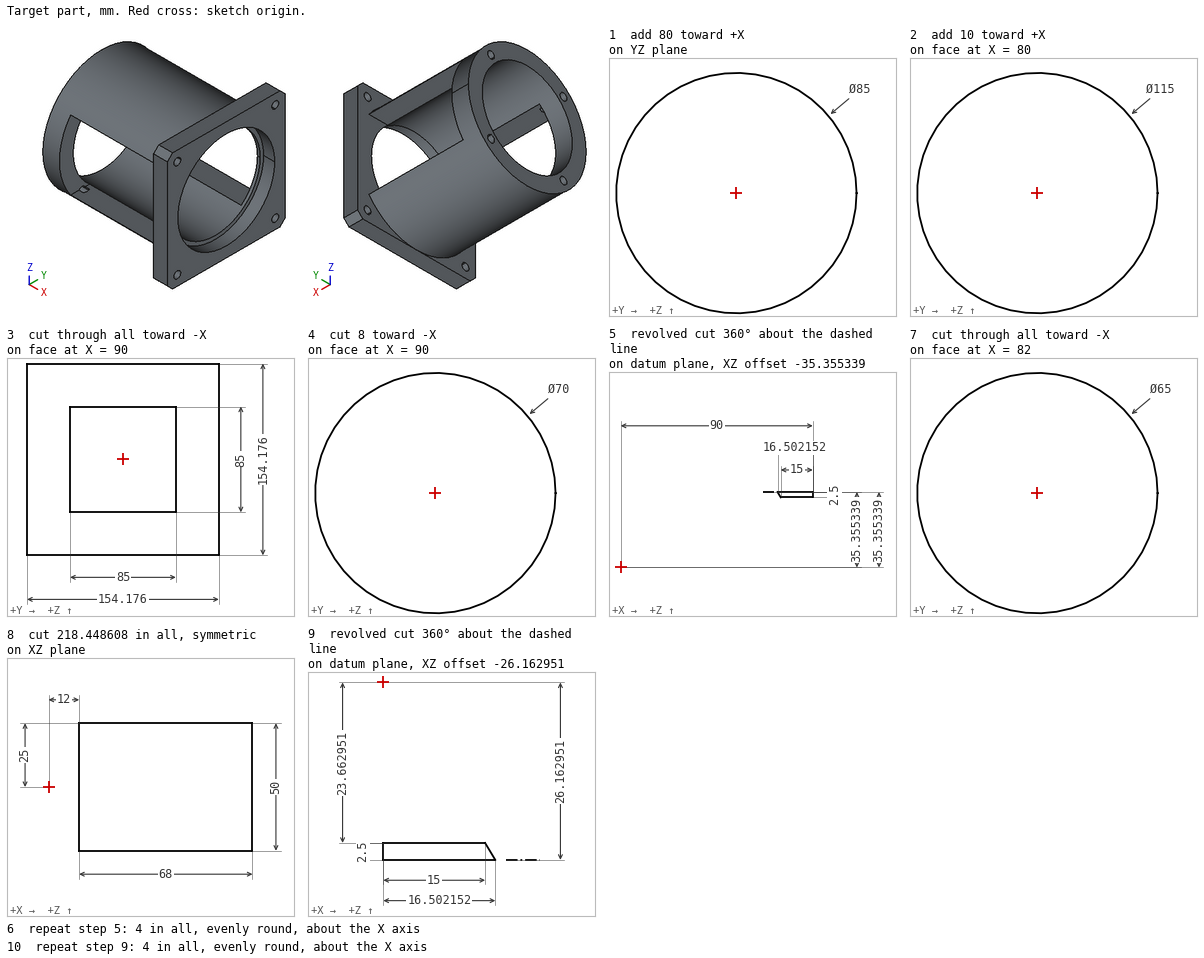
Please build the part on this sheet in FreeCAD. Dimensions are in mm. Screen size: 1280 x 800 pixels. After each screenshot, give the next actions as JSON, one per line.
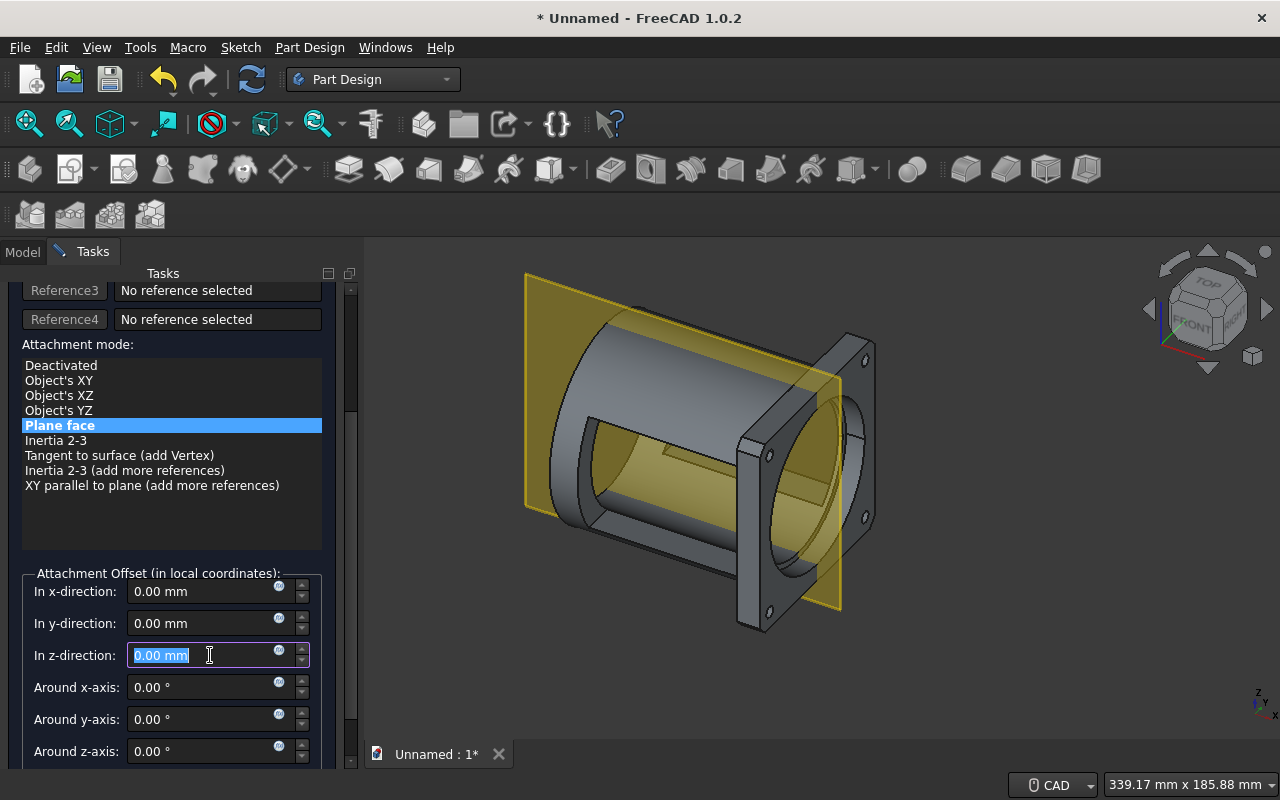
{"action": "type", "text": "-26.162951"}
{"action": "key", "text": "Tab"}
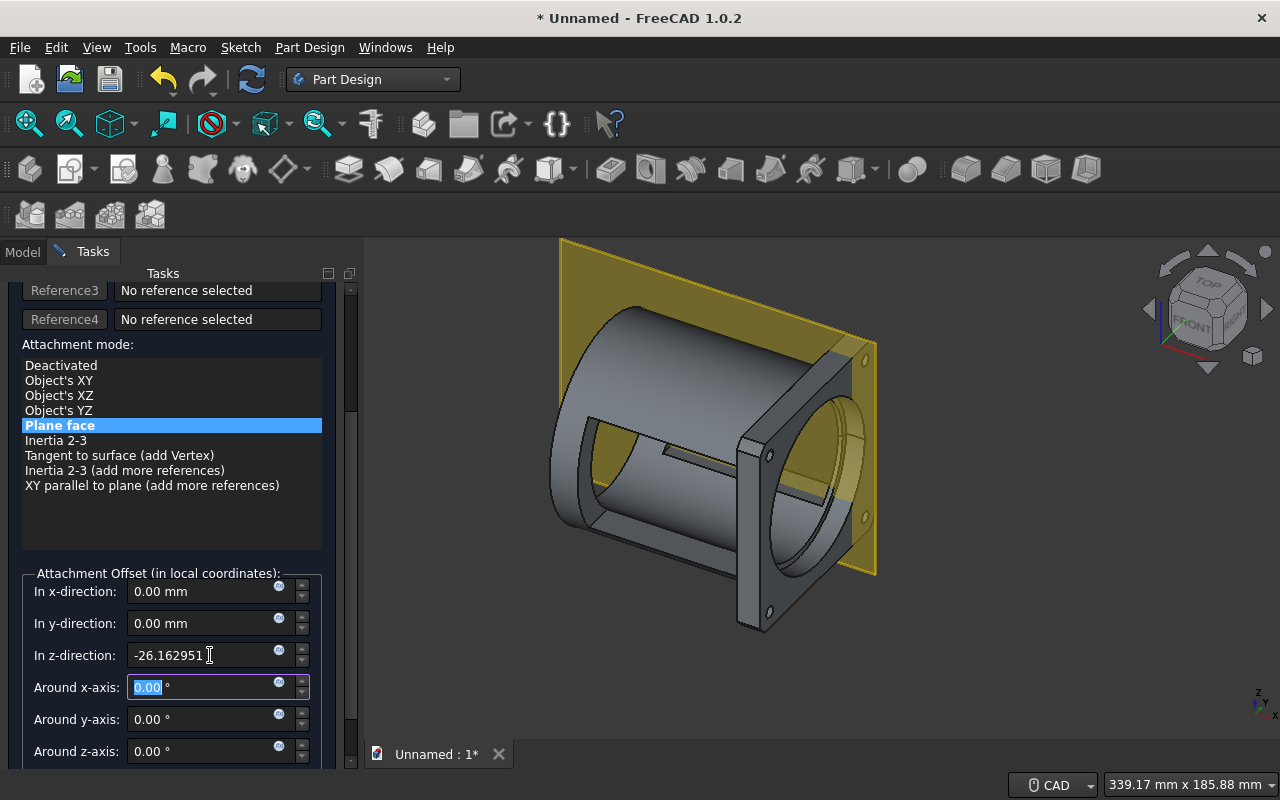
{"action": "scroll", "coordinate": [351, 526], "scroll_direction": "up", "scroll_amount": 4}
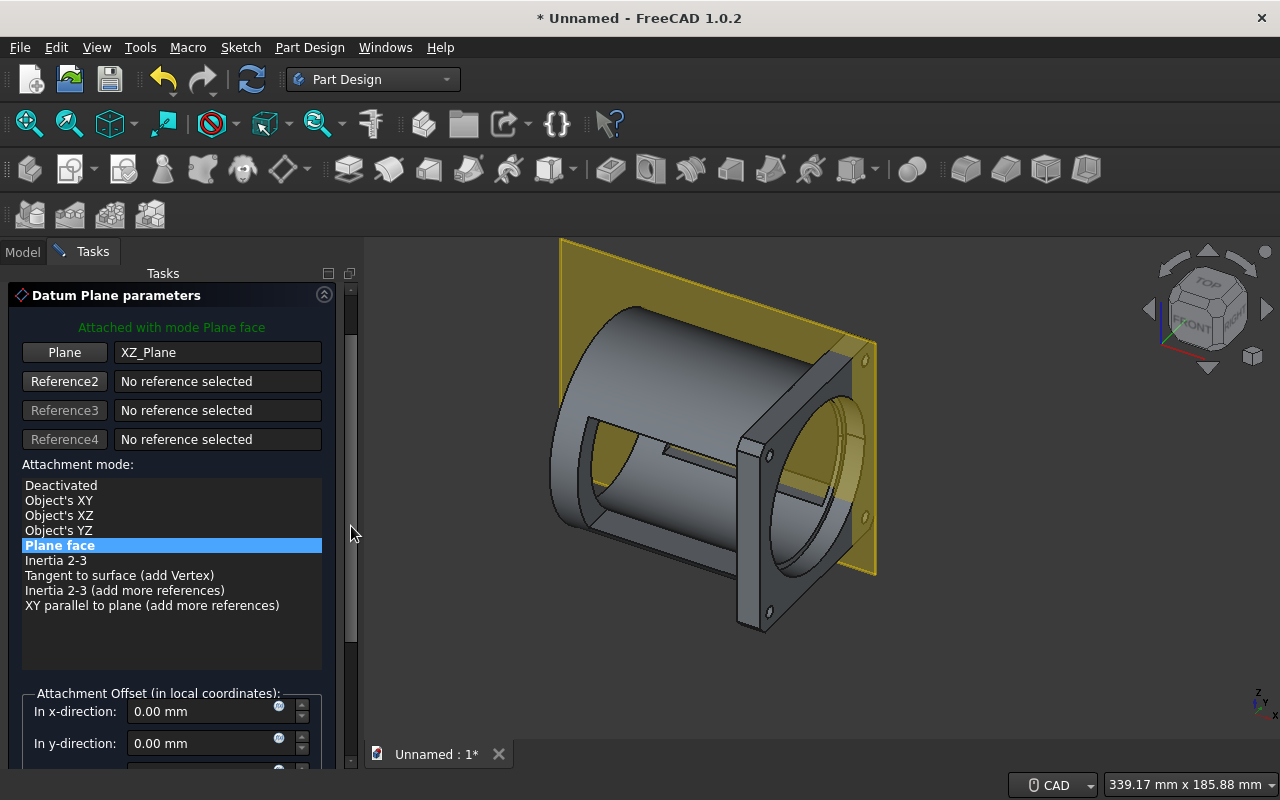
{"action": "left_click", "coordinate": [124, 312]}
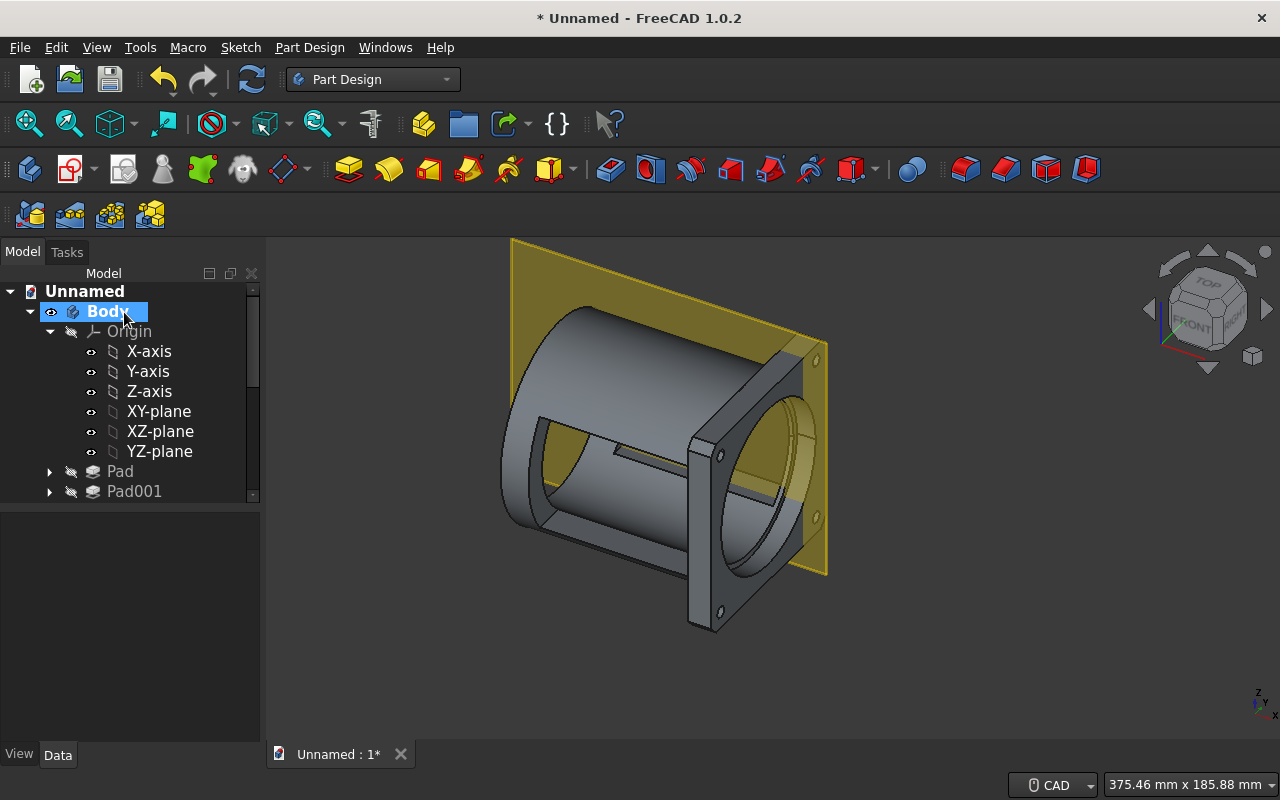
{"action": "scroll", "coordinate": [100, 387], "scroll_direction": "down", "scroll_amount": 3}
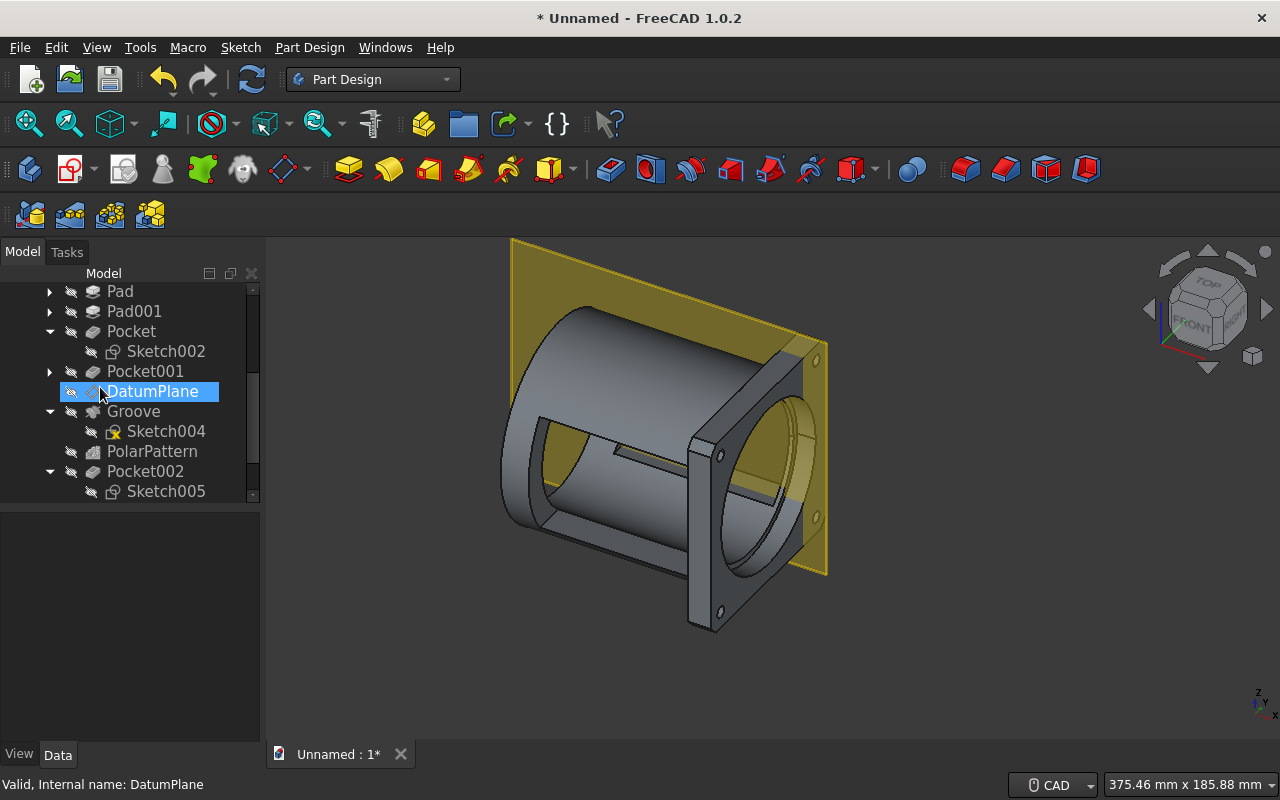
{"action": "scroll", "coordinate": [140, 387], "scroll_direction": "up", "scroll_amount": 15}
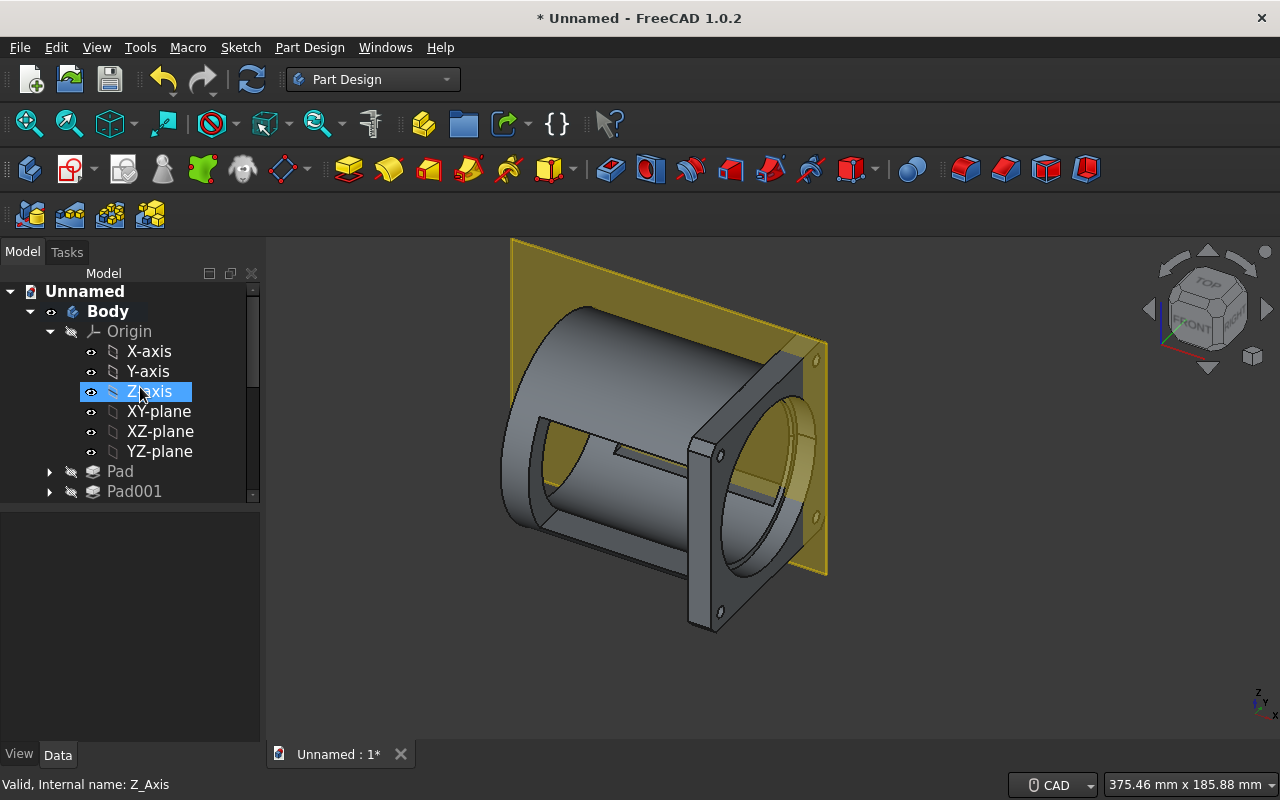
{"action": "scroll", "coordinate": [100, 387], "scroll_direction": "down", "scroll_amount": 6}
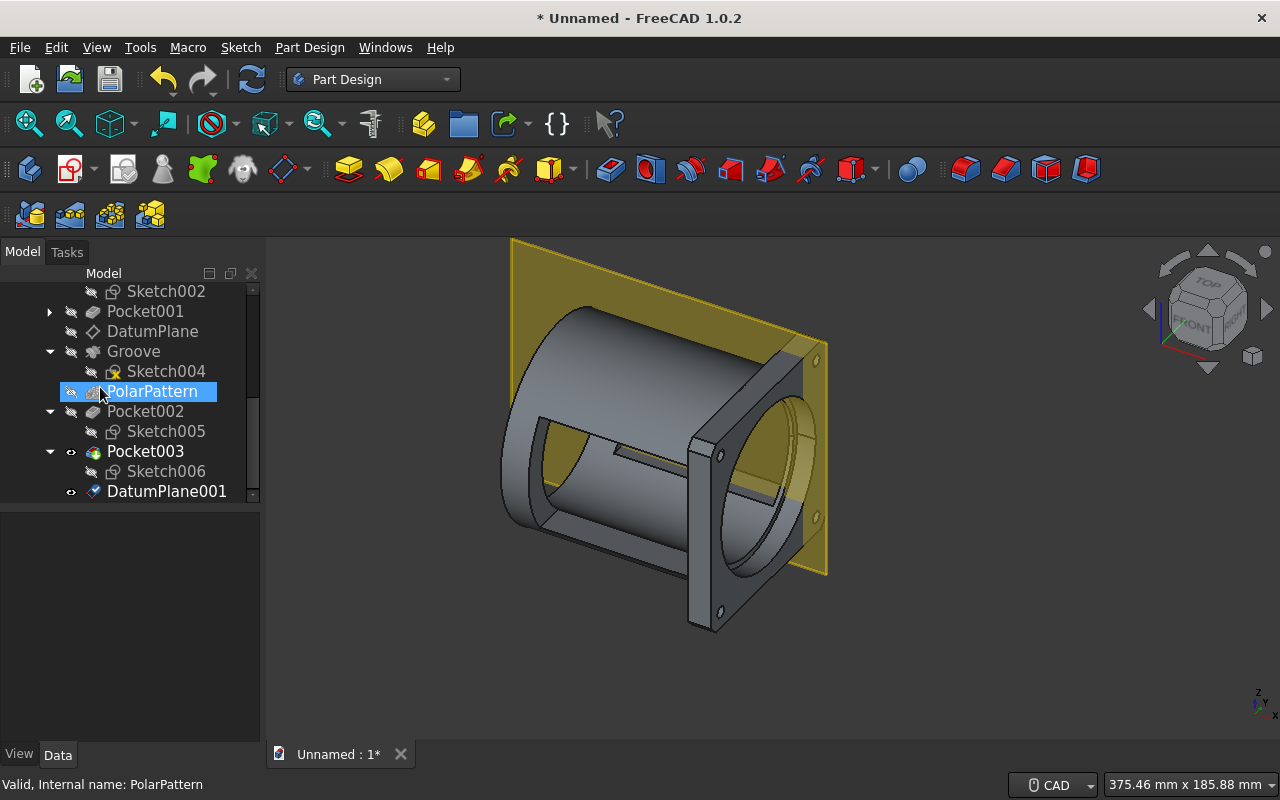
{"action": "left_click", "coordinate": [116, 492]}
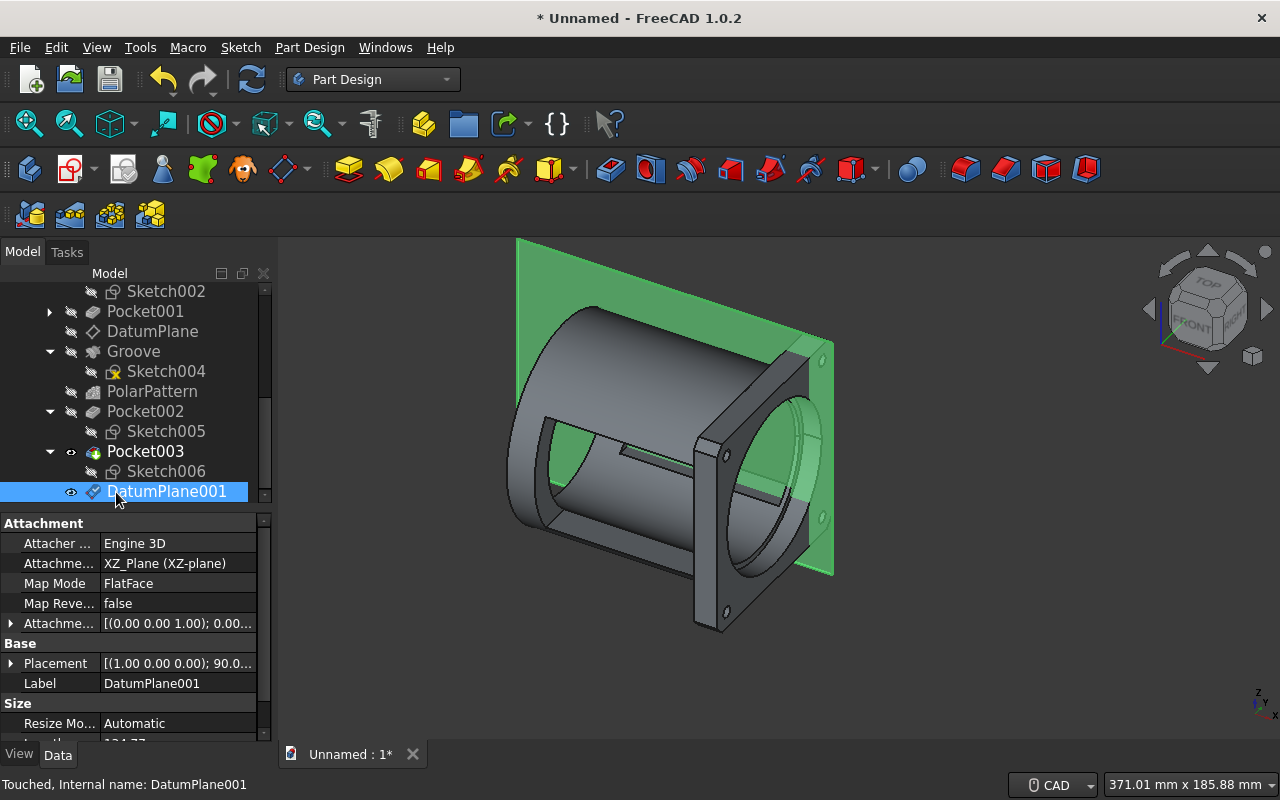
{"action": "left_click", "coordinate": [70, 170]}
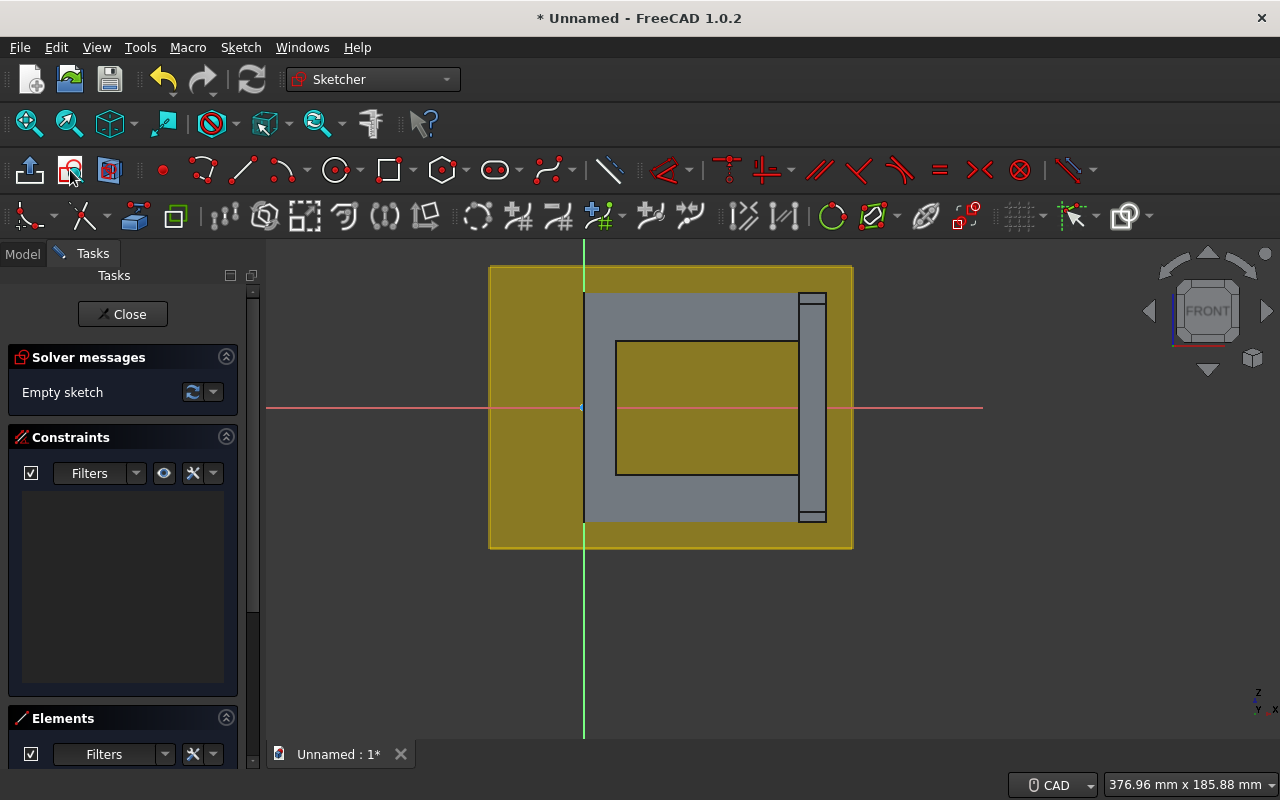
{"action": "left_click", "coordinate": [110, 170]}